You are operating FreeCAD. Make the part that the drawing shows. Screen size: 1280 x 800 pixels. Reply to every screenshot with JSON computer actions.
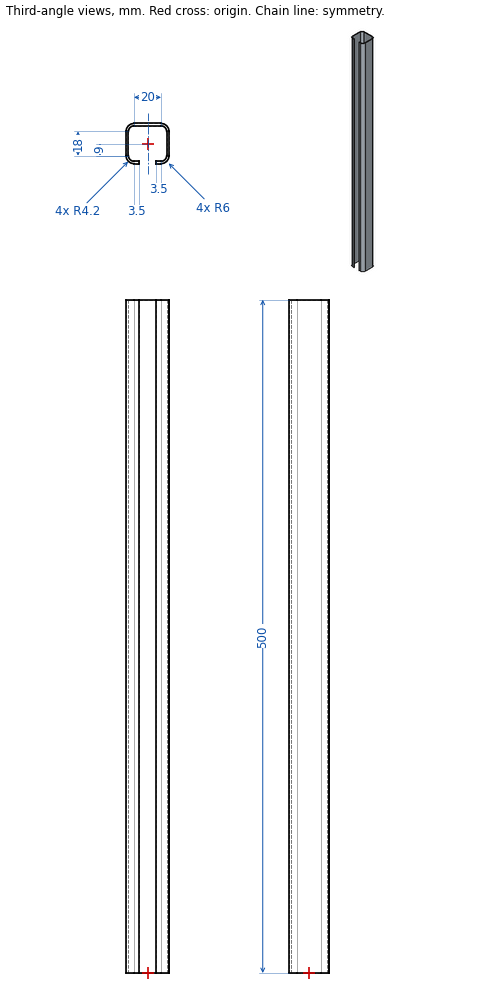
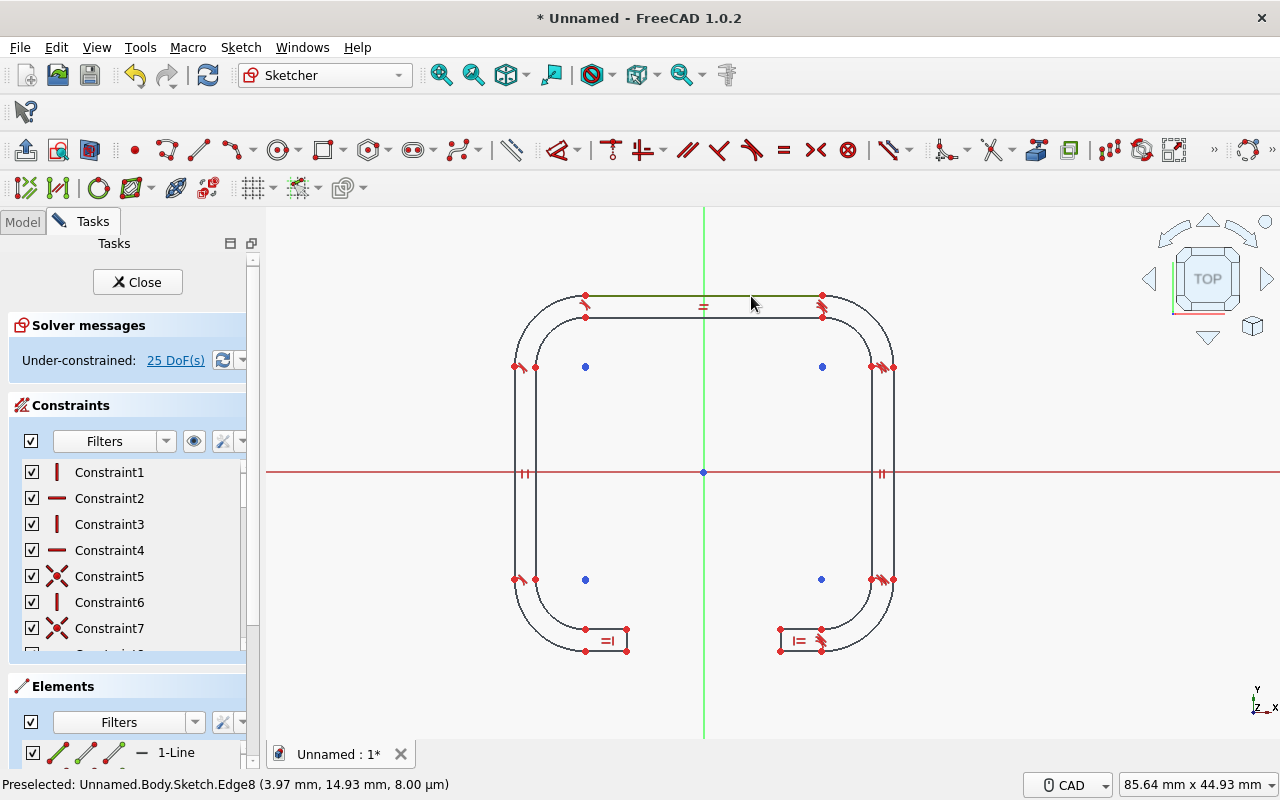
{"action": "left_click", "coordinate": [554, 303]}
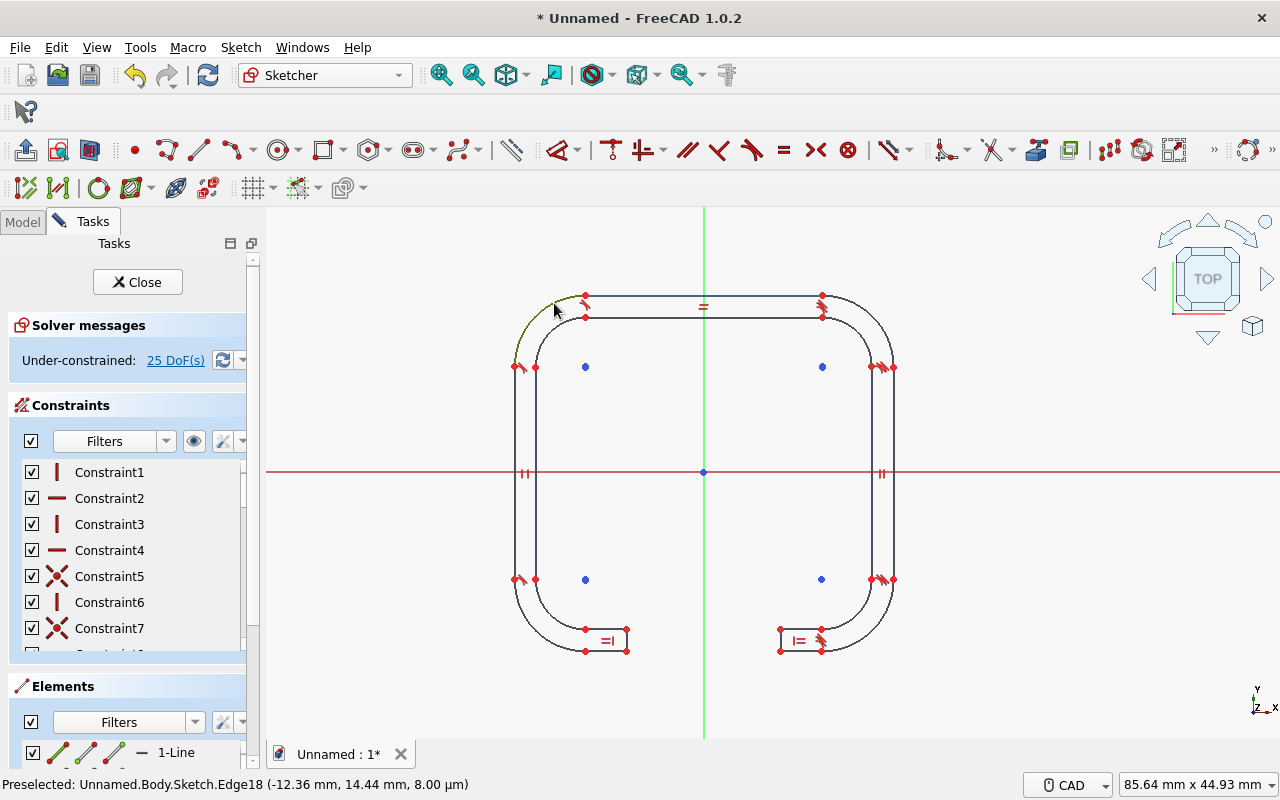
{"action": "left_click", "coordinate": [752, 150]}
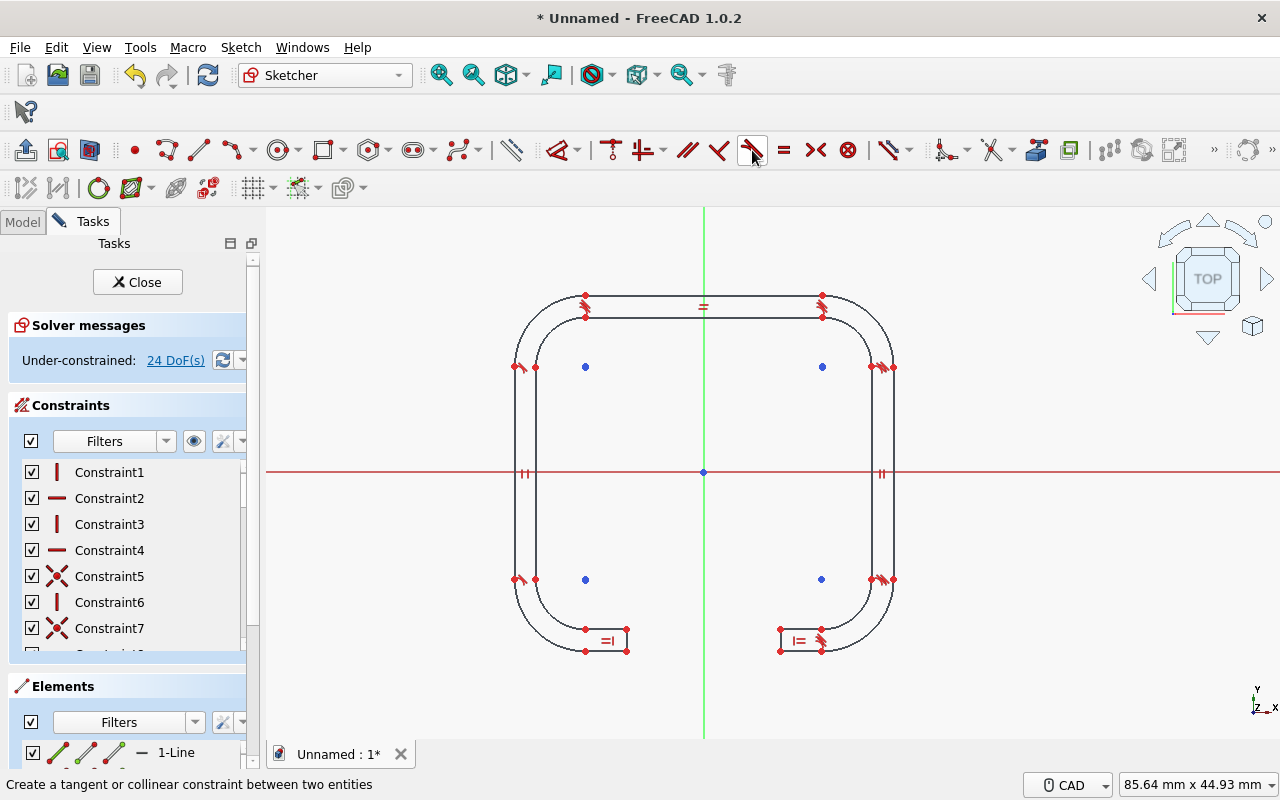
{"action": "left_click", "coordinate": [515, 430]}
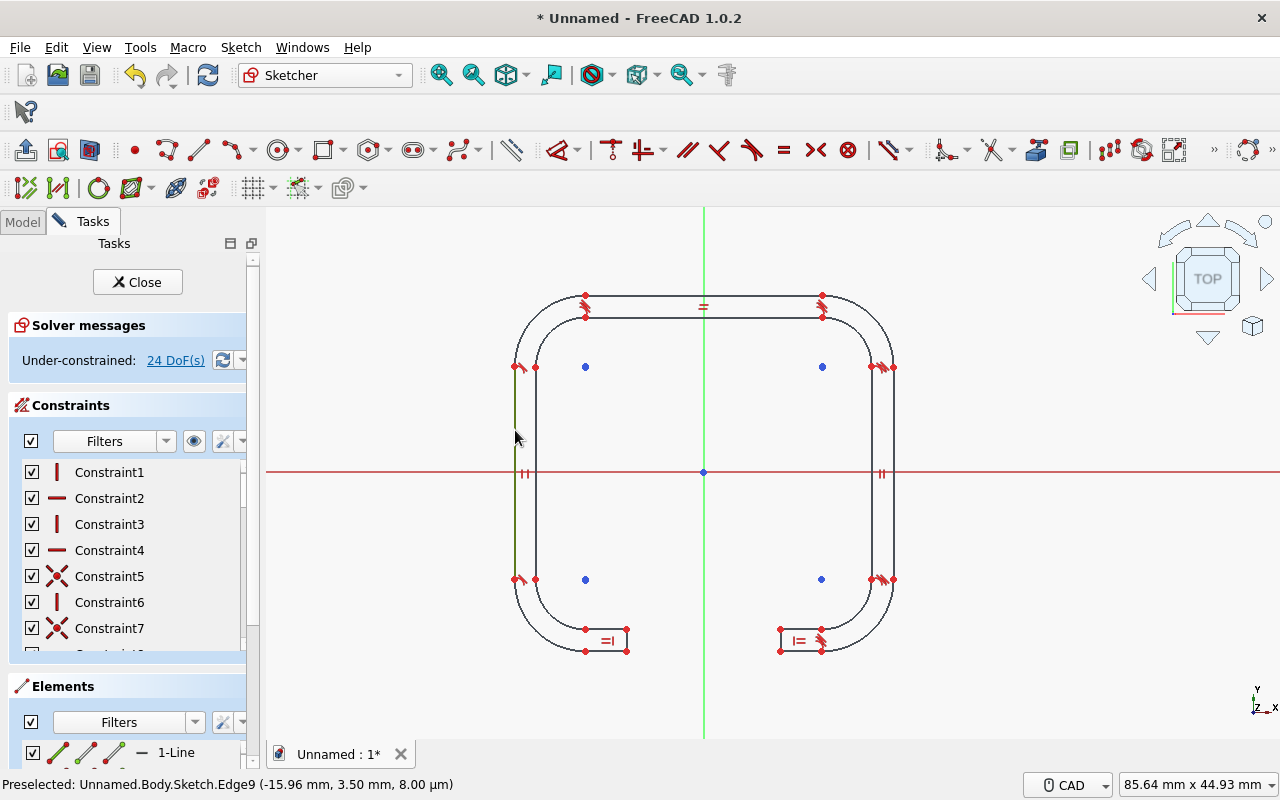
{"action": "left_click", "coordinate": [554, 303]}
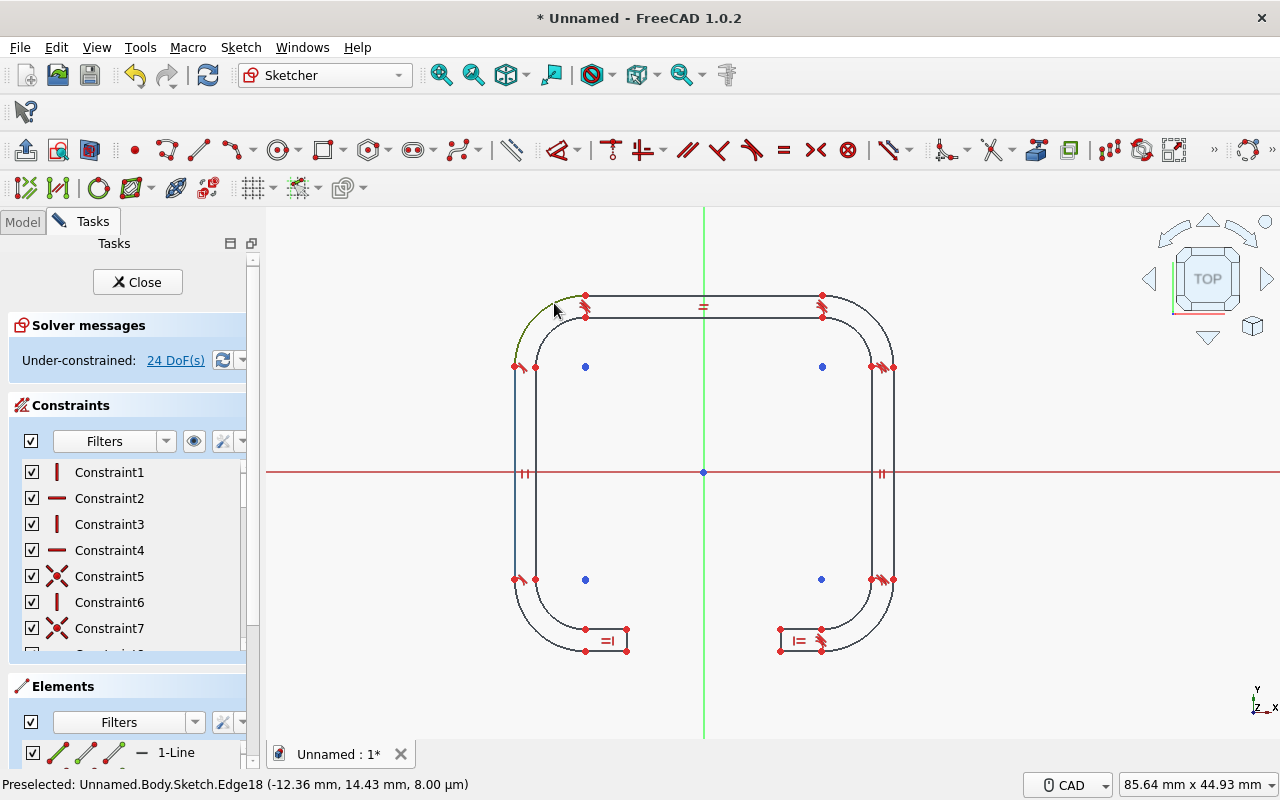
{"action": "left_click", "coordinate": [752, 150]}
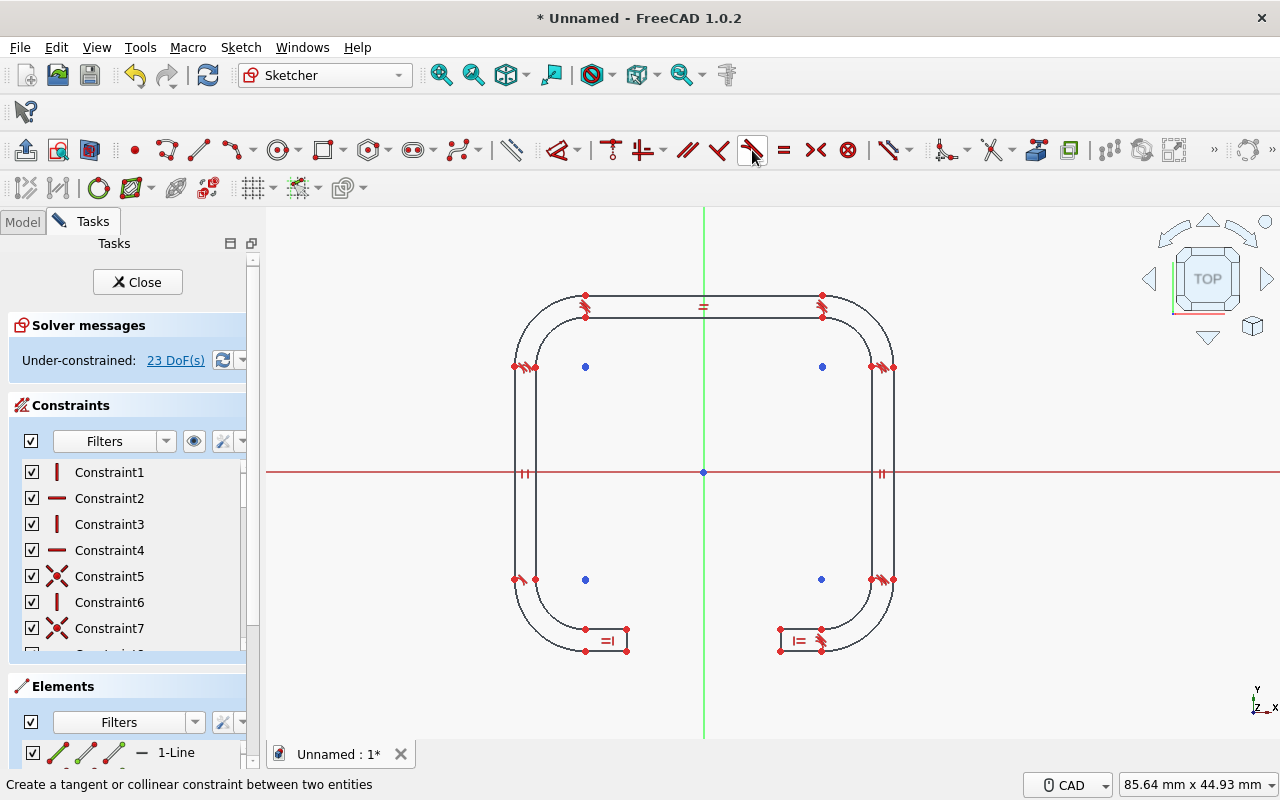
{"action": "left_click", "coordinate": [515, 430]}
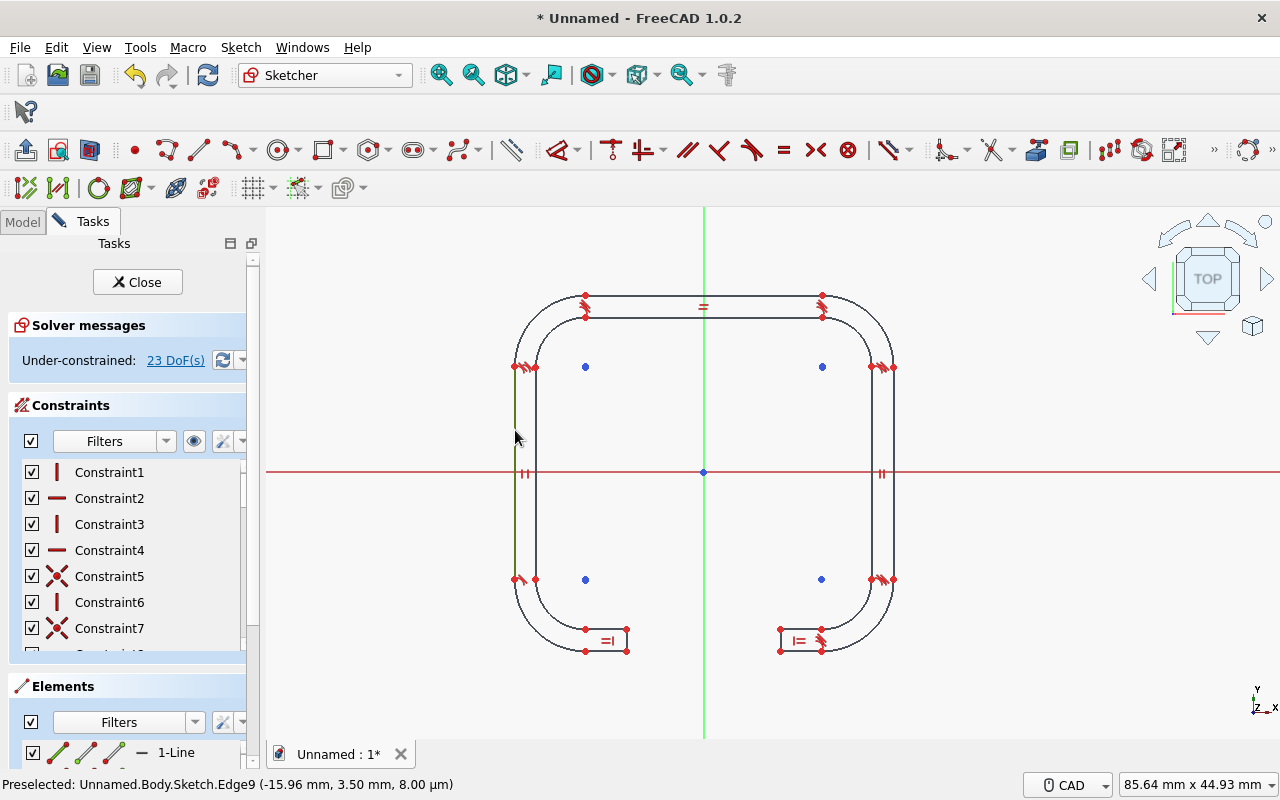
{"action": "left_click", "coordinate": [522, 612]}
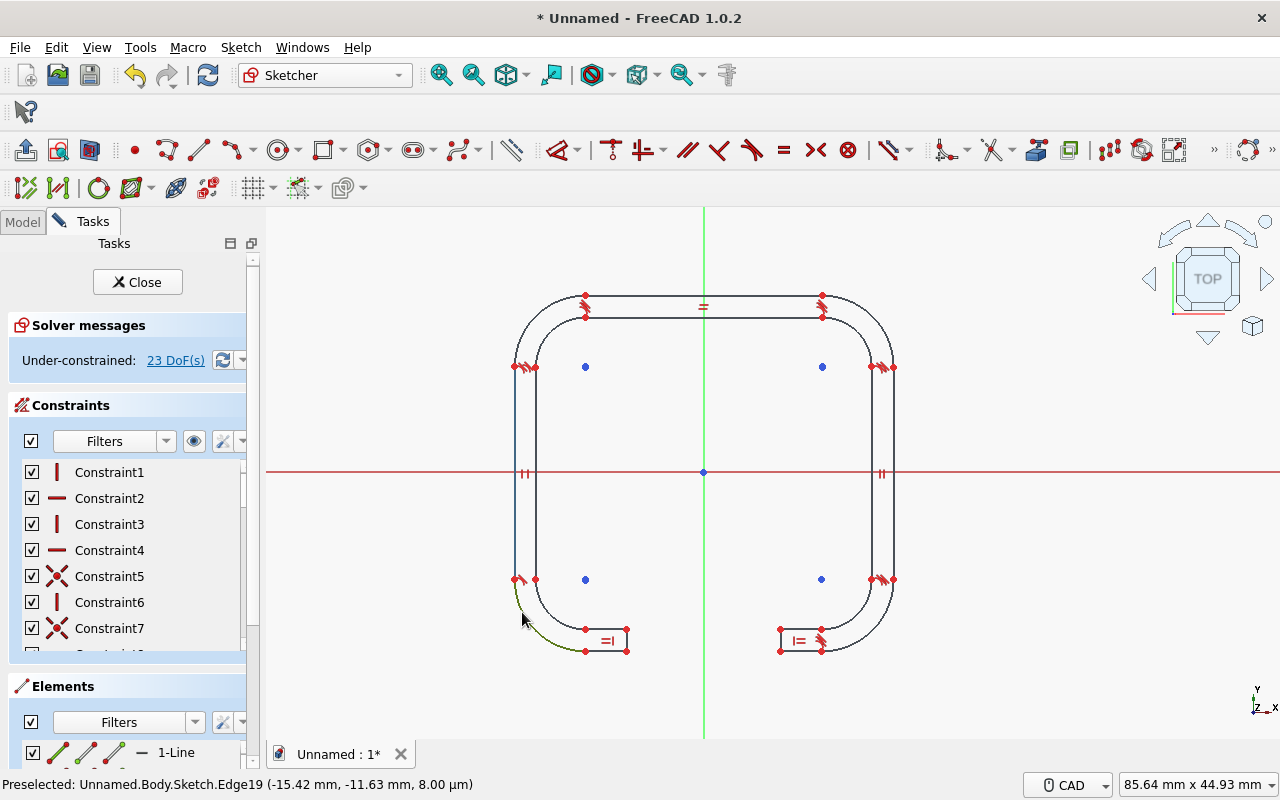
{"action": "left_click", "coordinate": [752, 150]}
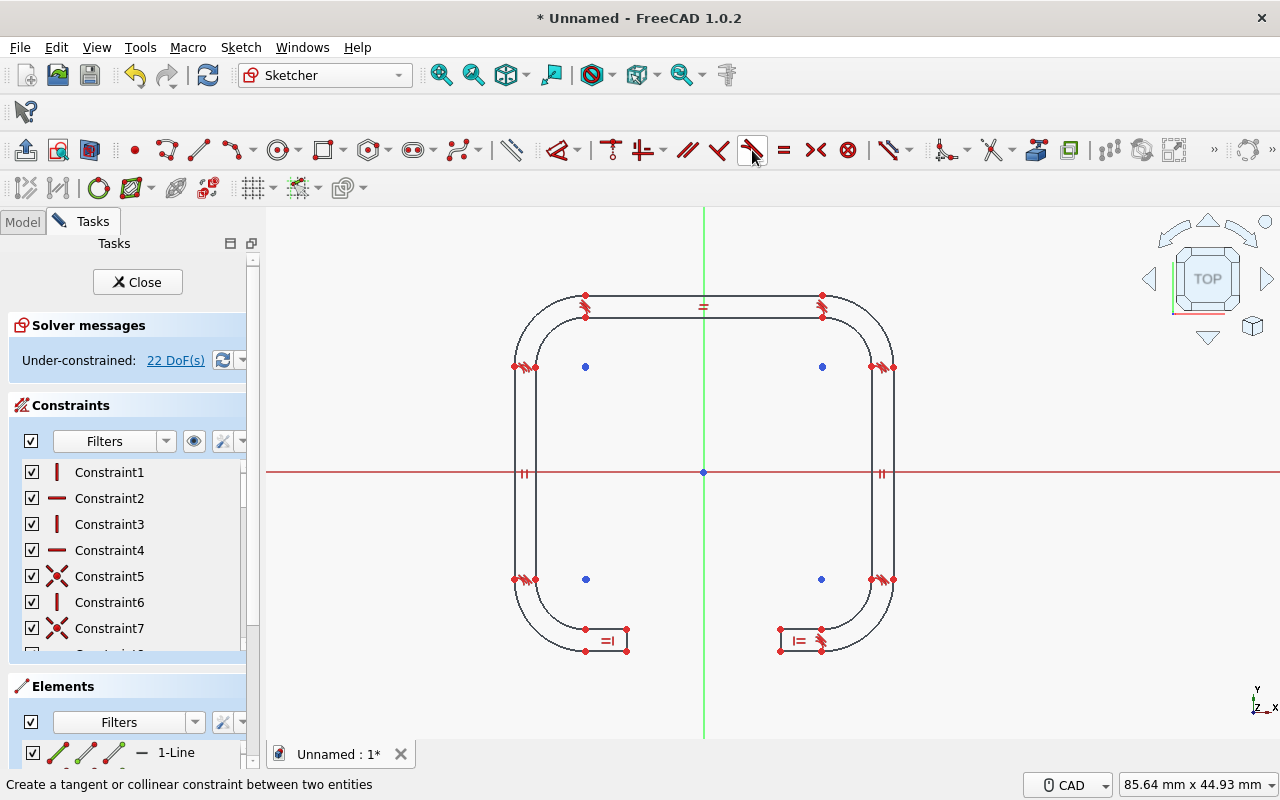
{"action": "left_click", "coordinate": [598, 651]}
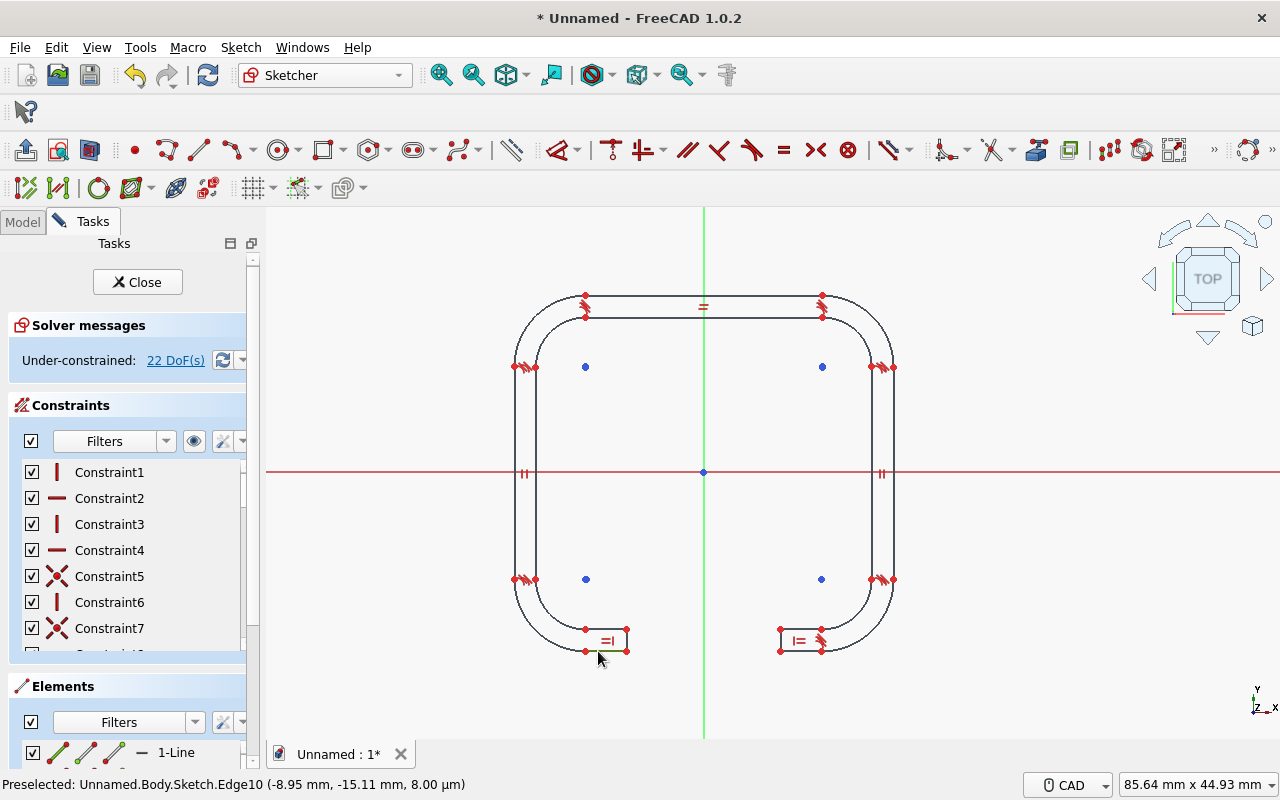
{"action": "left_click", "coordinate": [522, 612]}